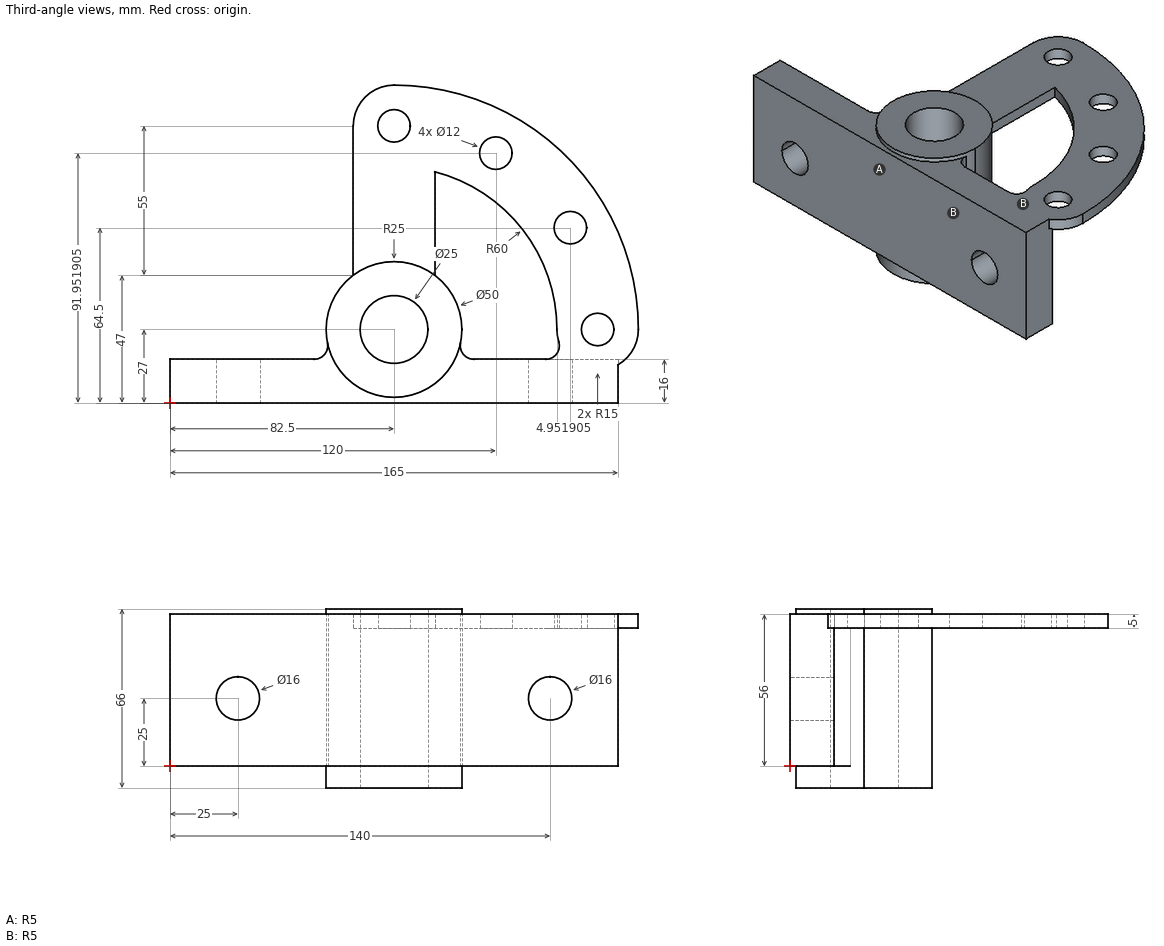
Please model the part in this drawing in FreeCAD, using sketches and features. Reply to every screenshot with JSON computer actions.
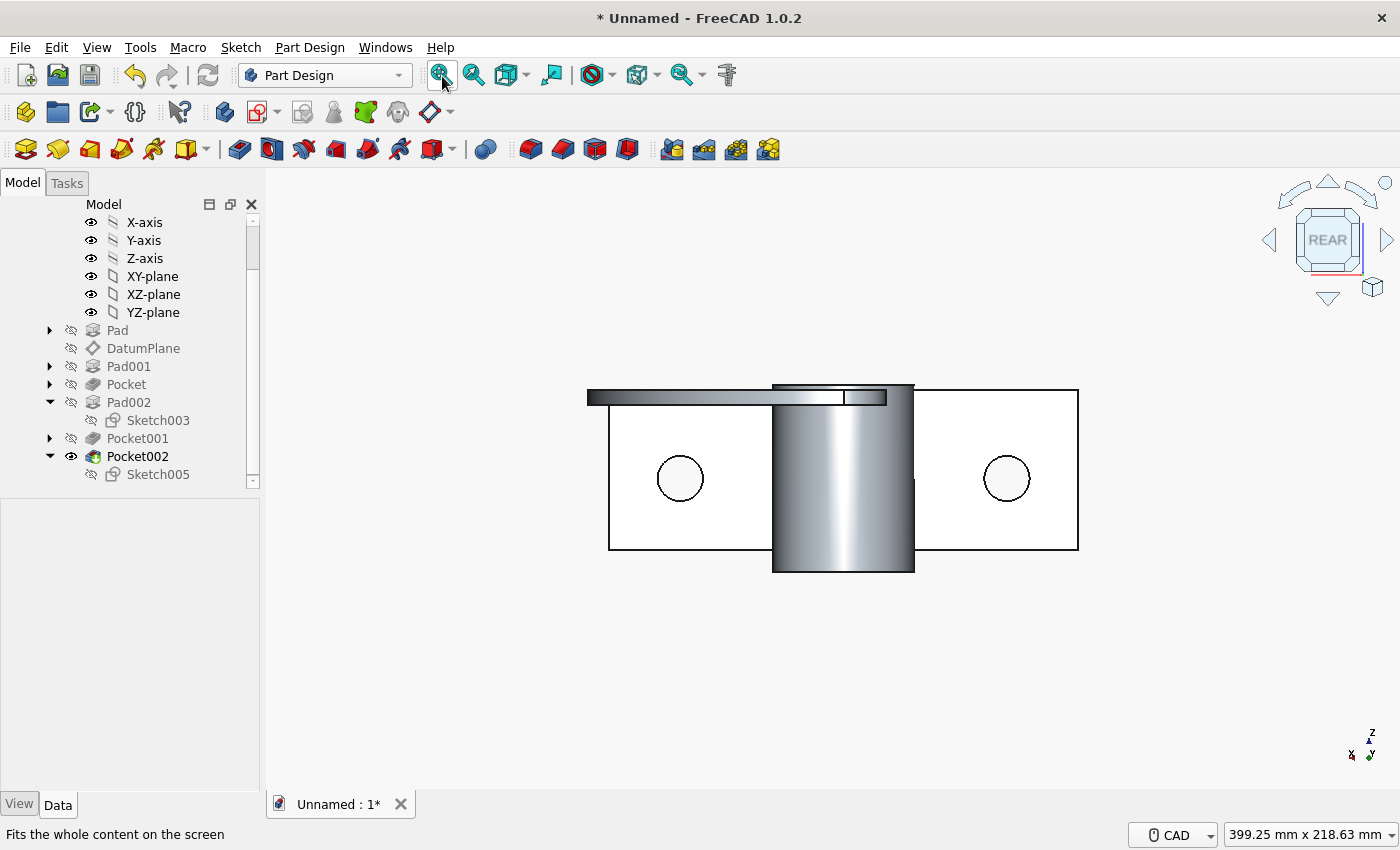
{"action": "key", "text": "0"}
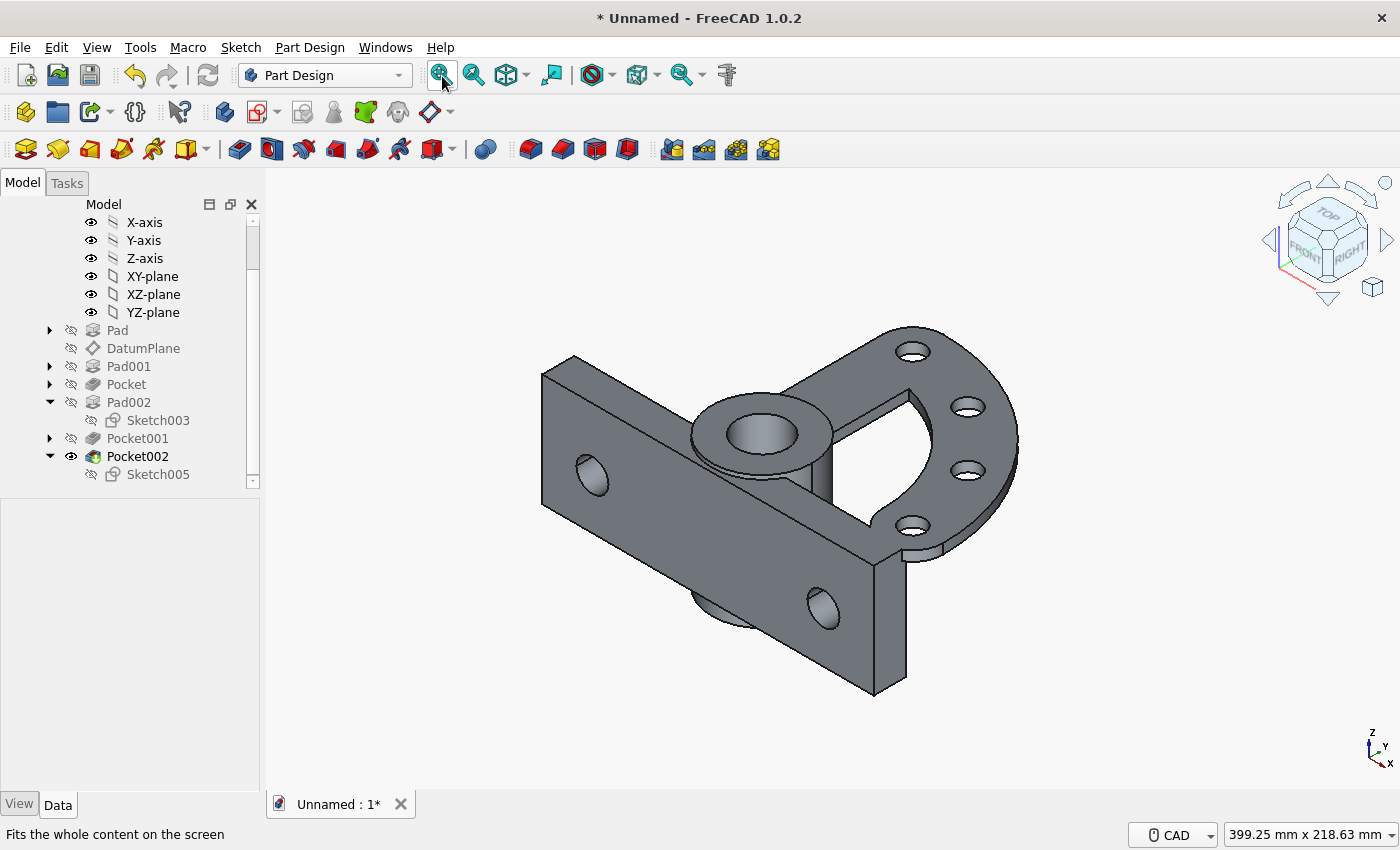
{"action": "key", "text": "2"}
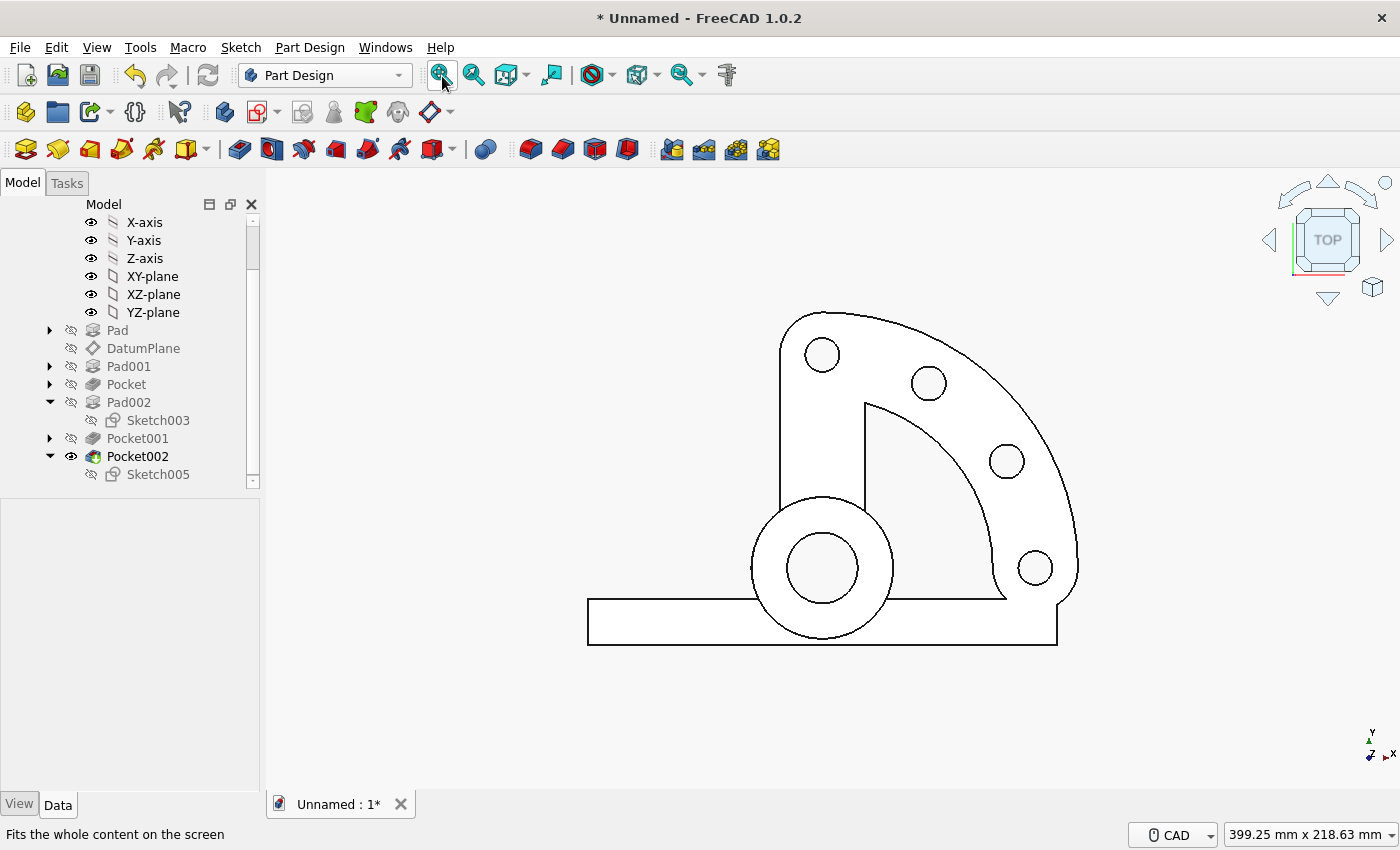
{"action": "key", "text": "1"}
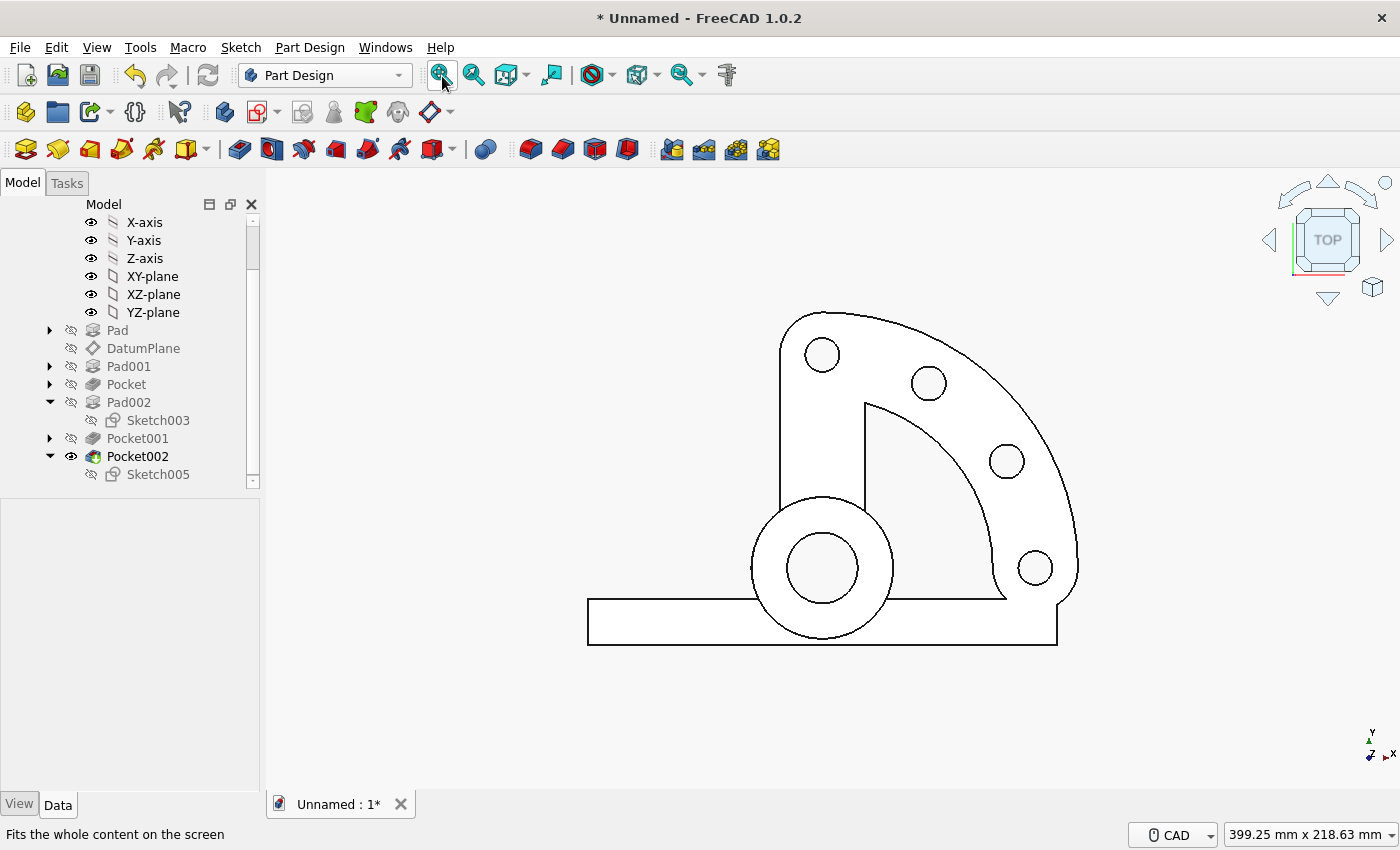
{"action": "left_click", "coordinate": [442, 76]}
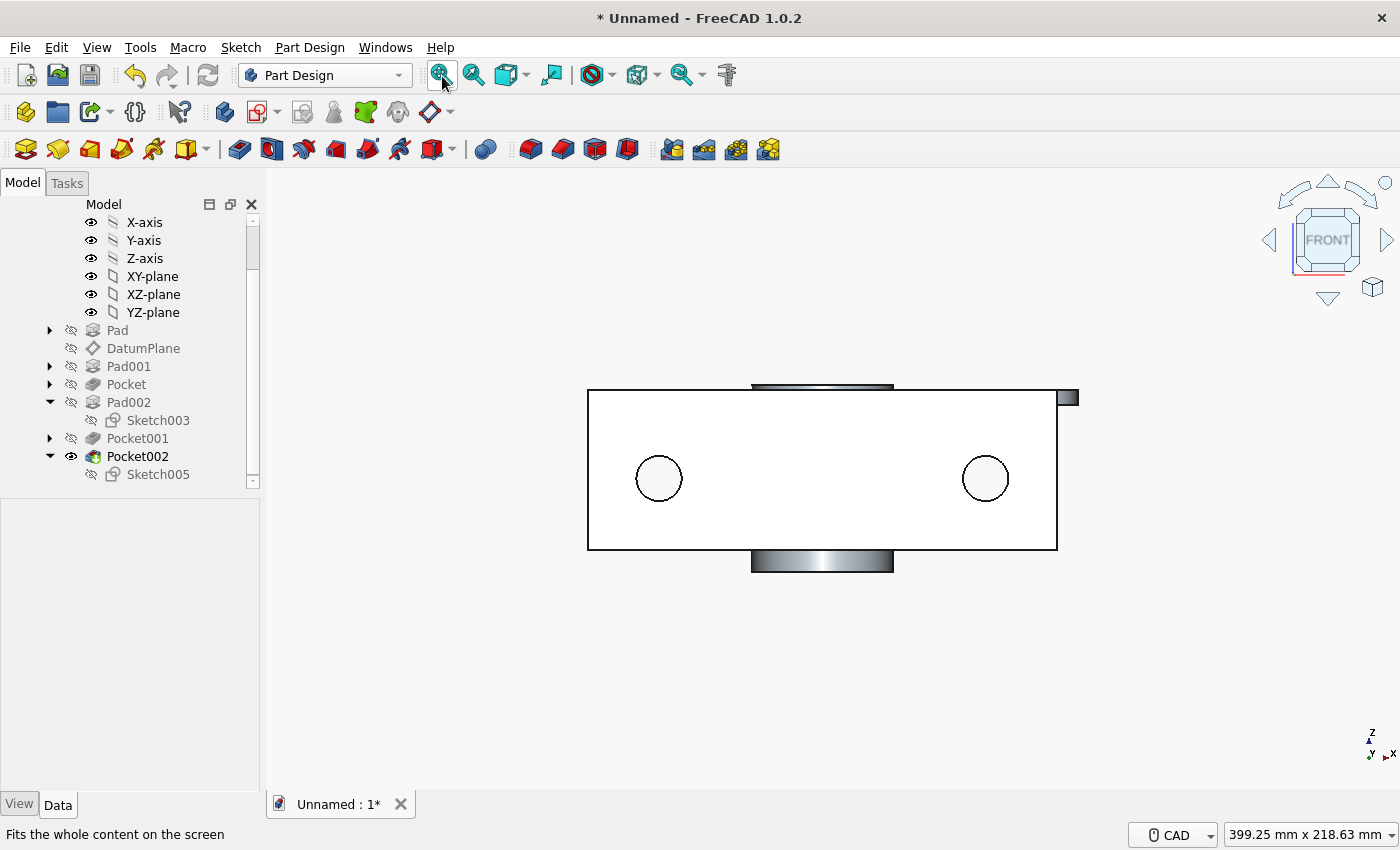
{"action": "key", "text": "3"}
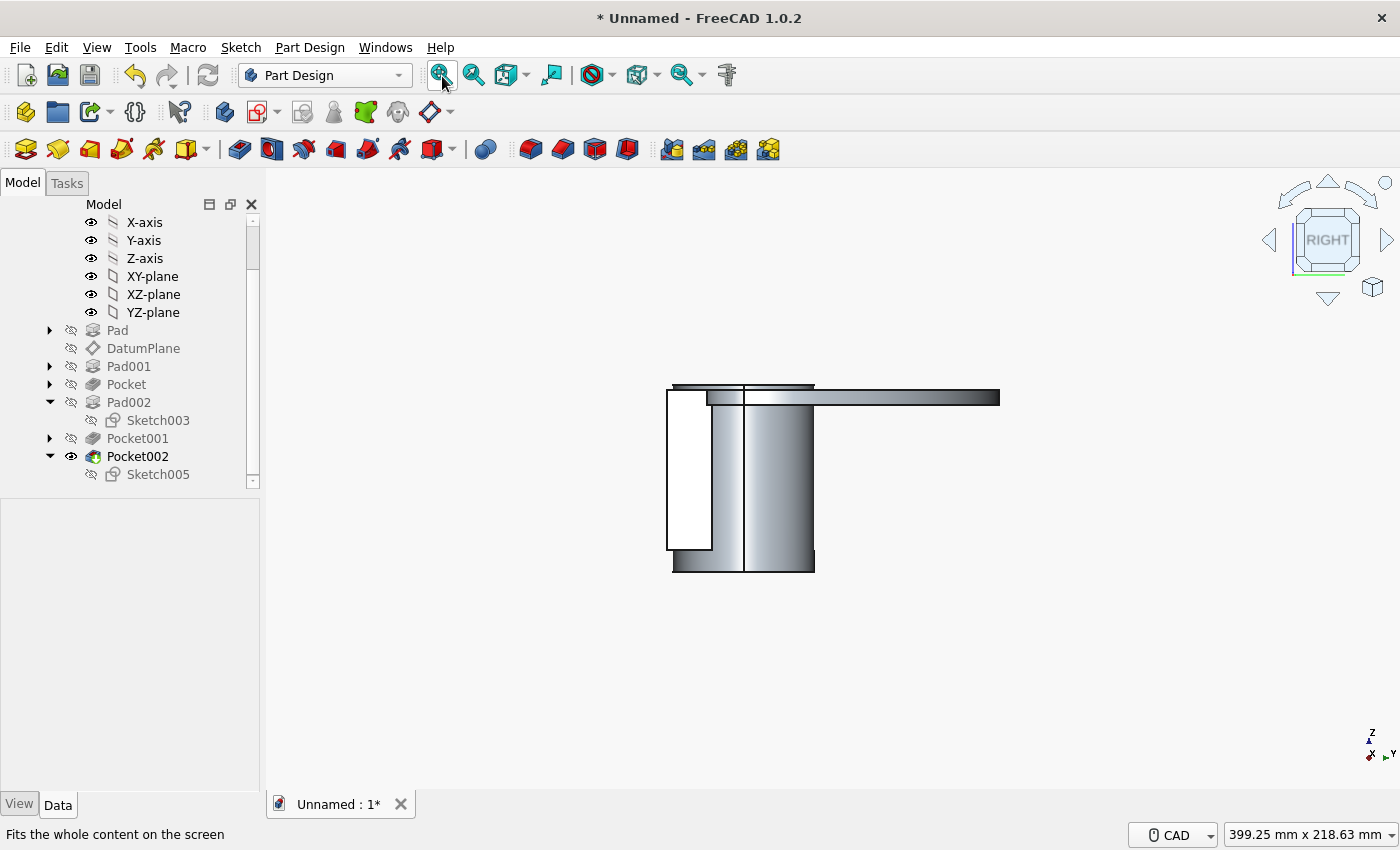
{"action": "left_click", "coordinate": [442, 76]}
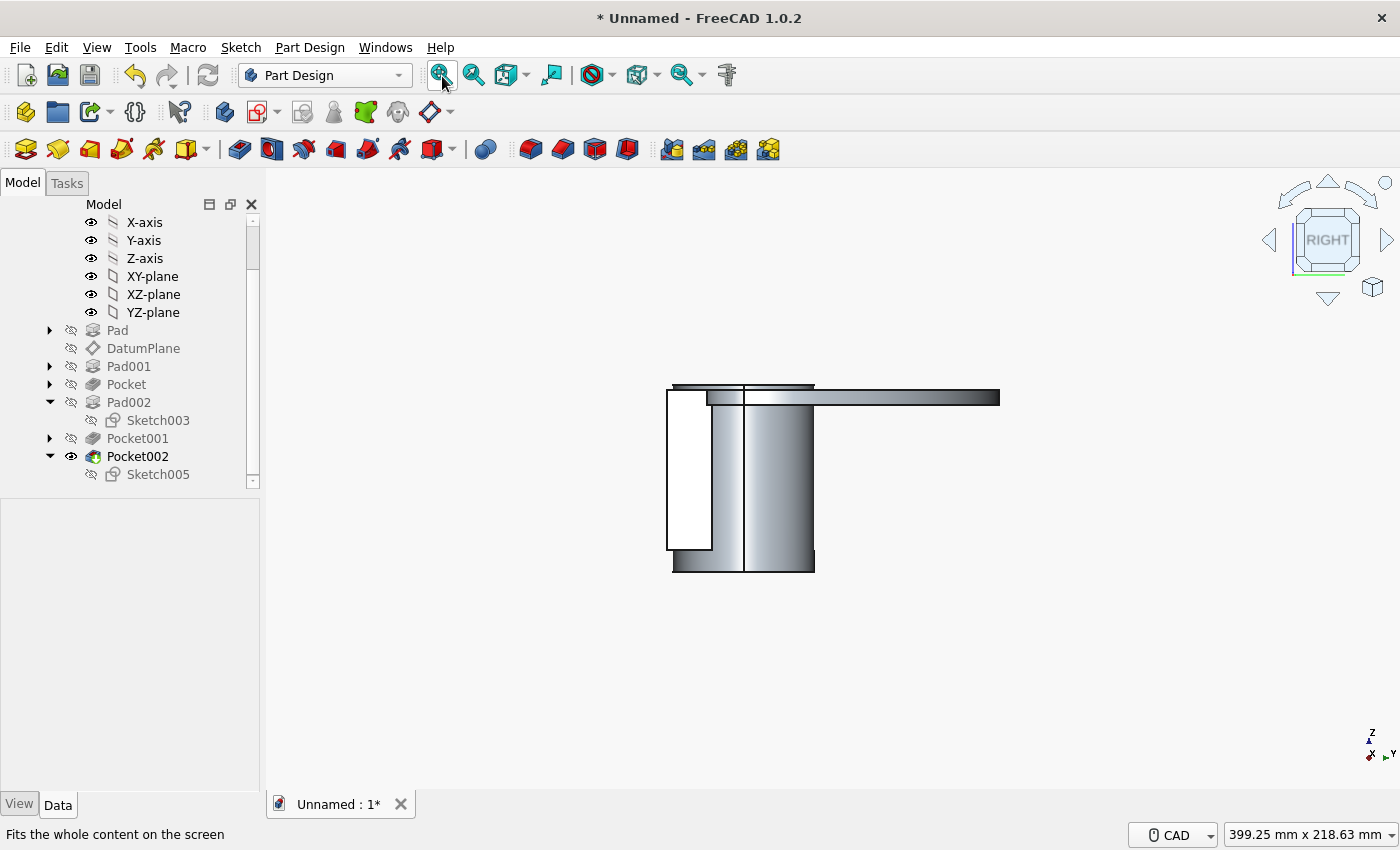
{"action": "key", "text": "5"}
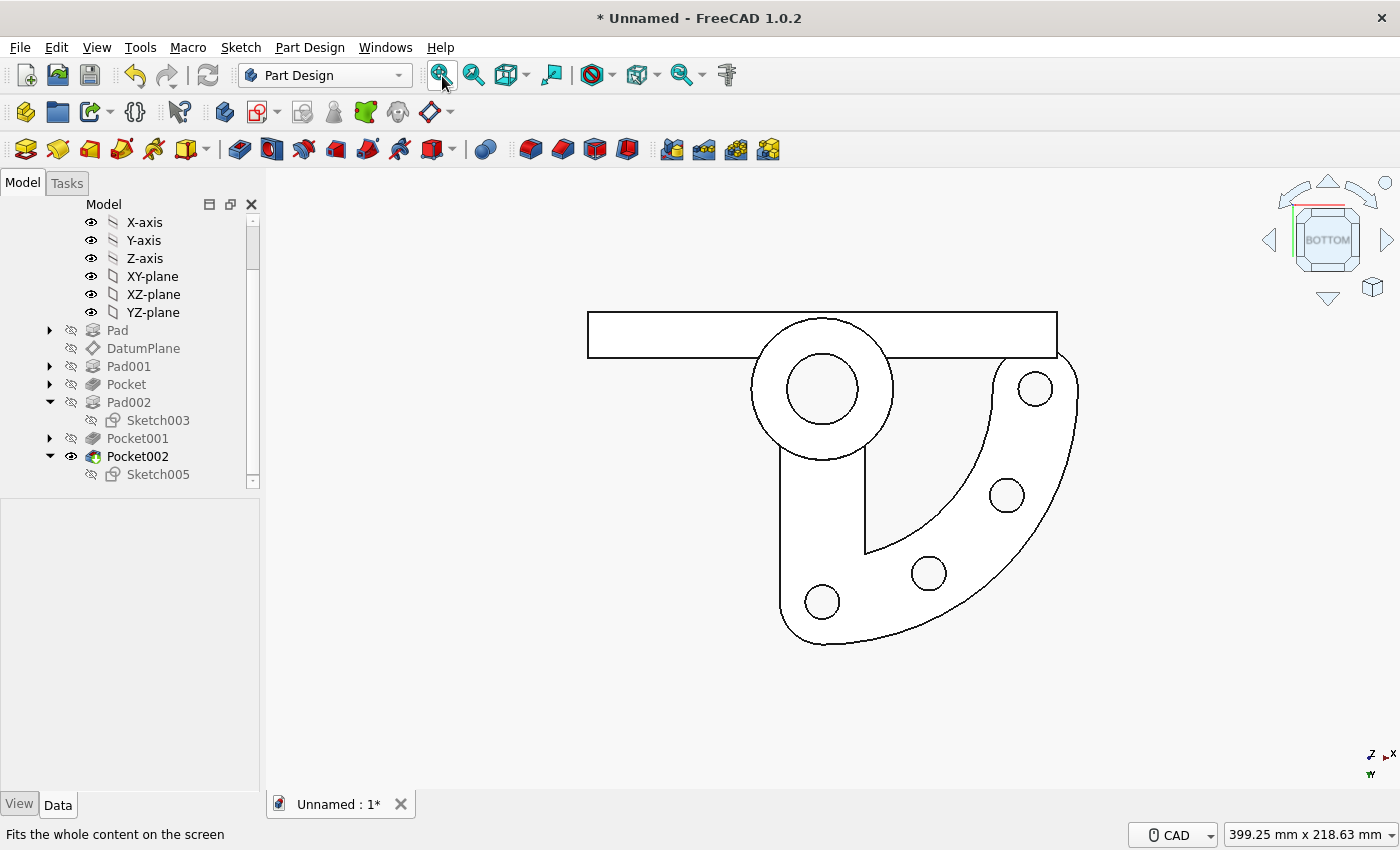
{"action": "key", "text": "4"}